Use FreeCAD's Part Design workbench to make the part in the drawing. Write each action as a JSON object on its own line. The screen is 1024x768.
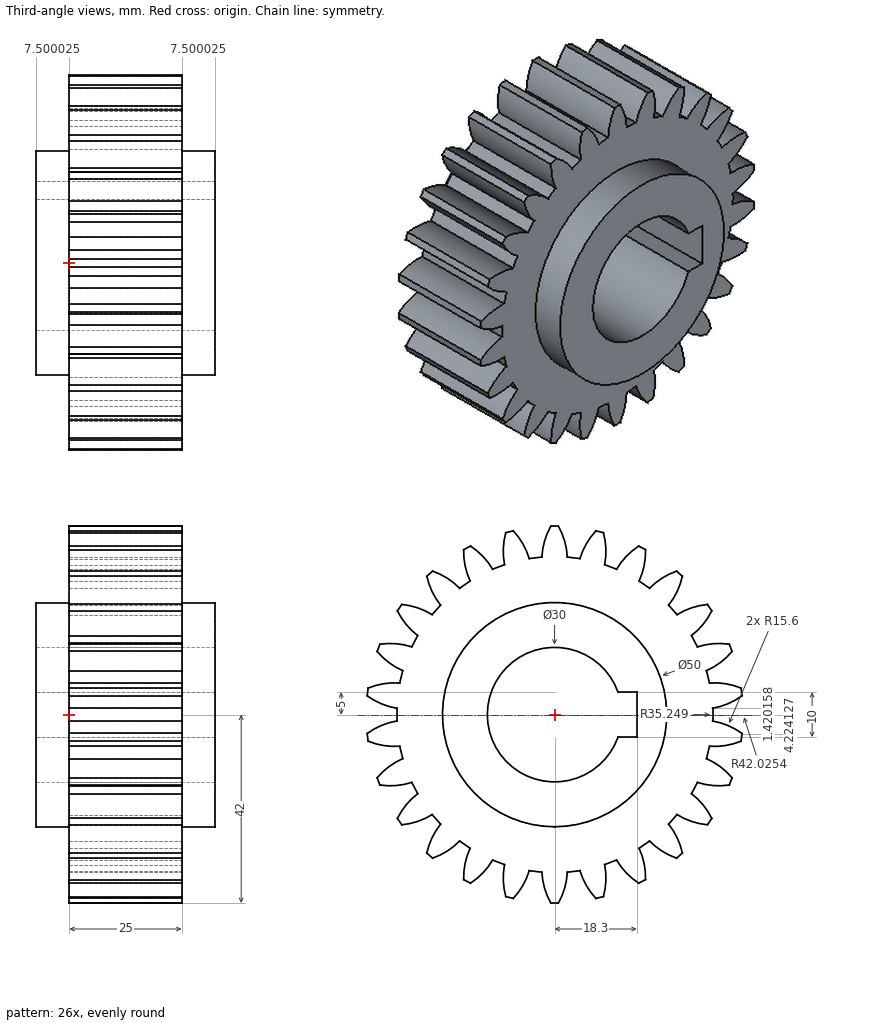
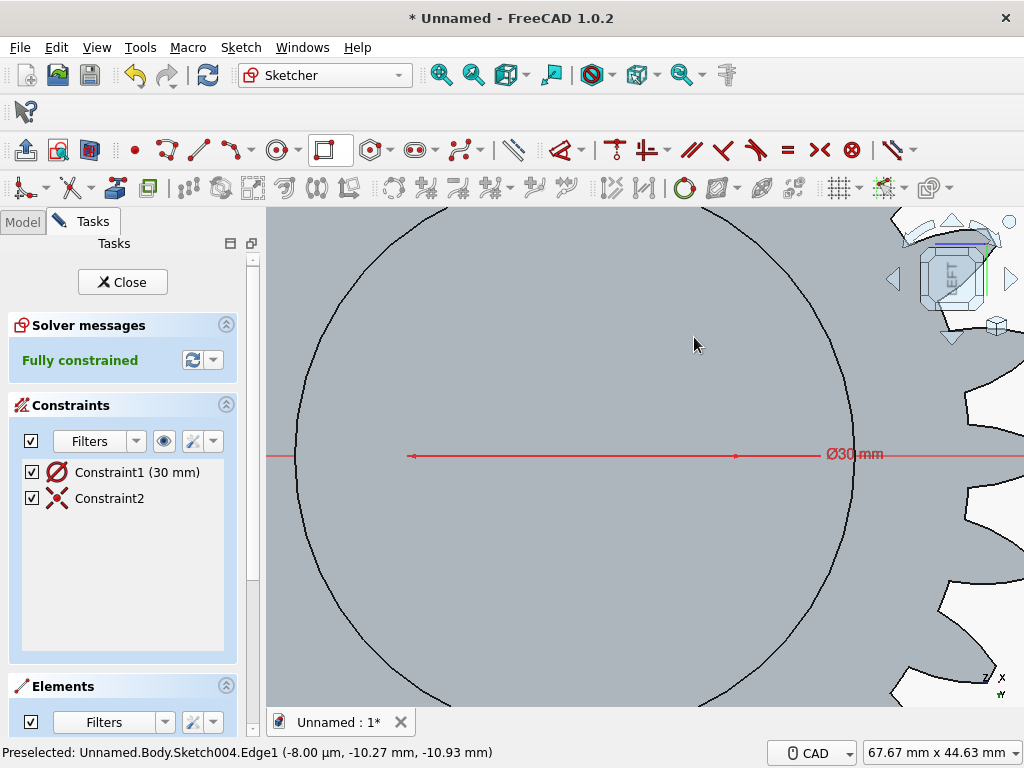
{"action": "left_click", "coordinate": [123, 282]}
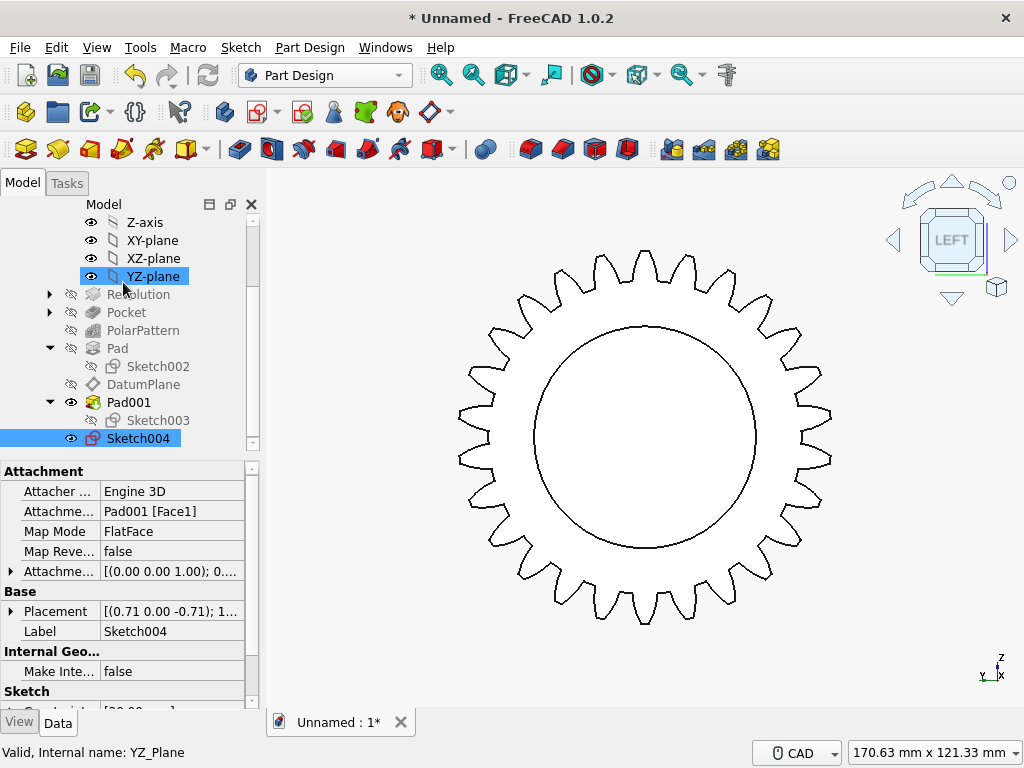
{"action": "left_click", "coordinate": [240, 150]}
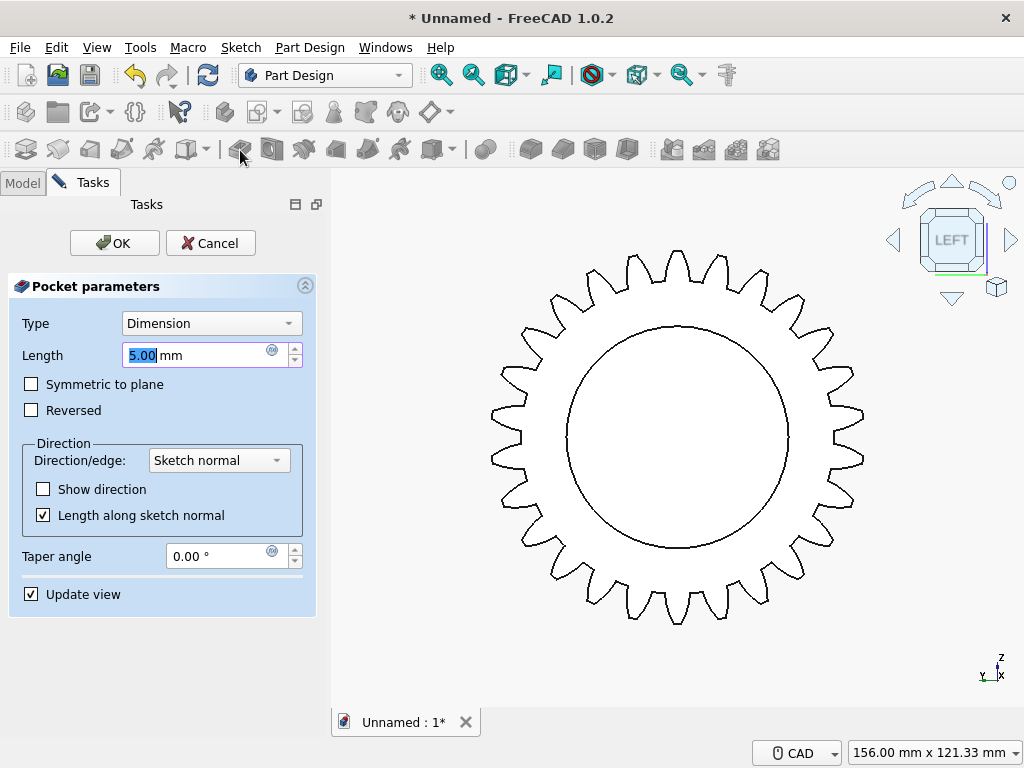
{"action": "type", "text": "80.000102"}
{"action": "key", "text": "Tab"}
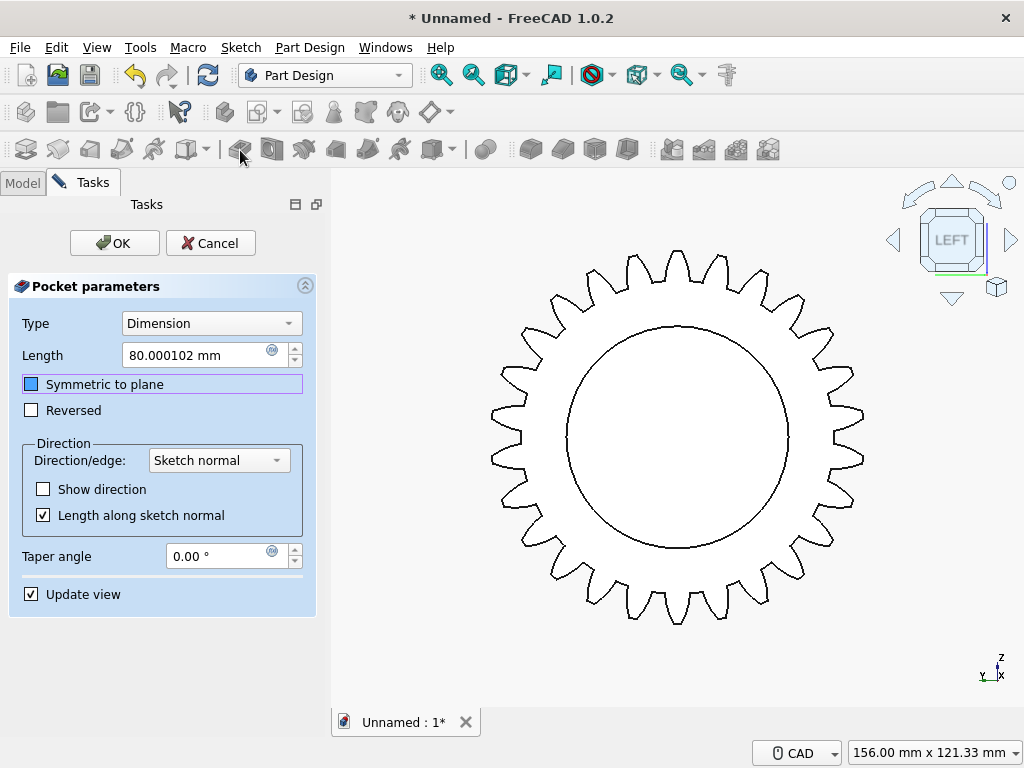
{"action": "left_click", "coordinate": [30, 384]}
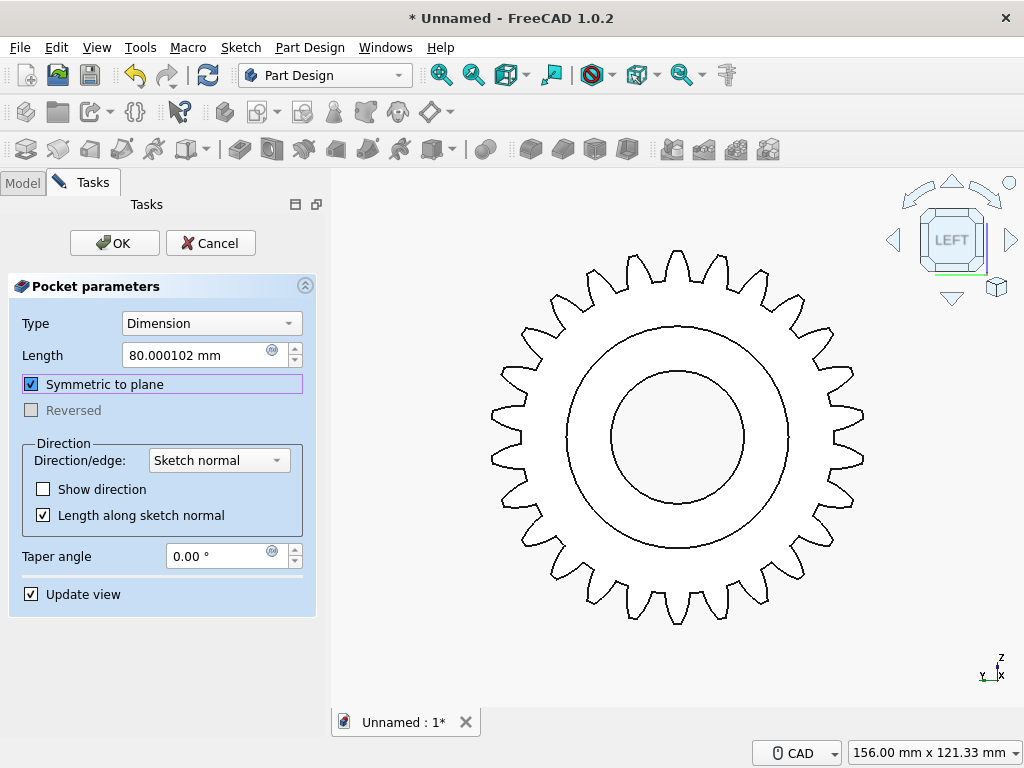
{"action": "left_click", "coordinate": [115, 243]}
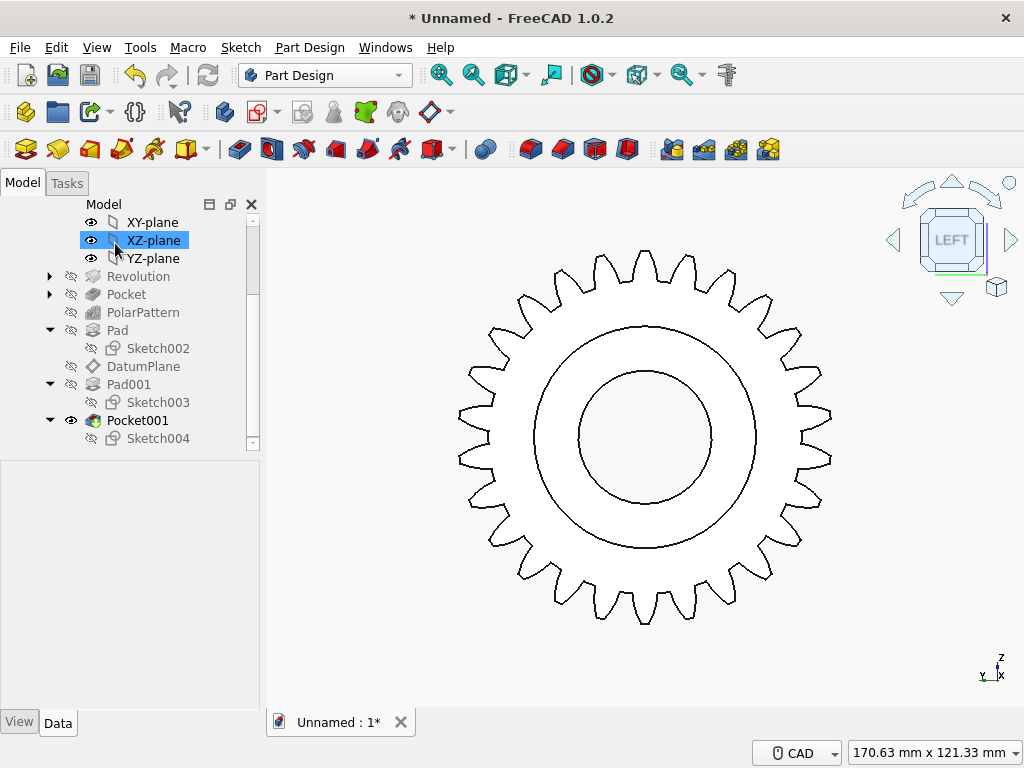
{"action": "left_click", "coordinate": [258, 112]}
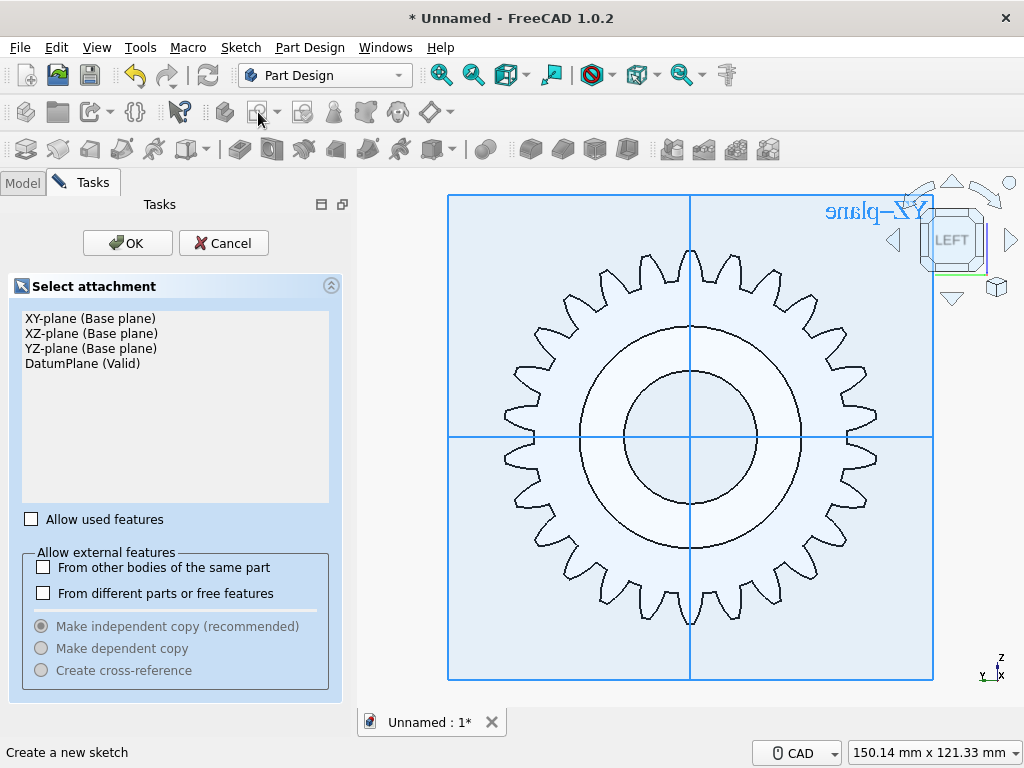
{"action": "left_click", "coordinate": [82, 348]}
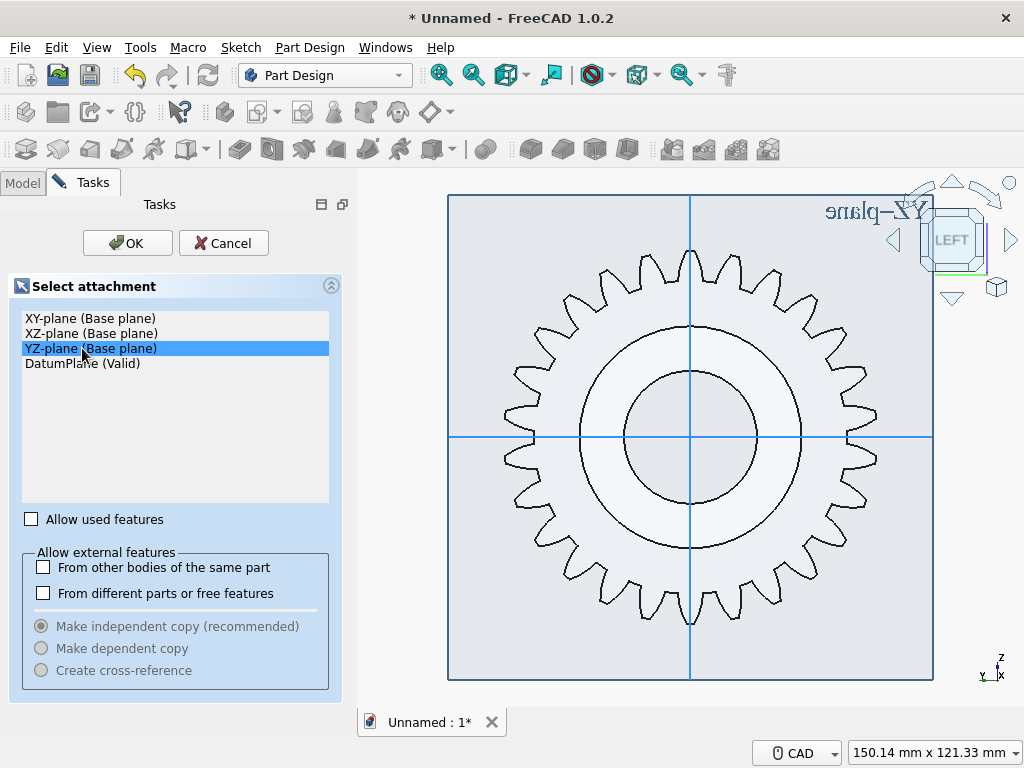
{"action": "left_click", "coordinate": [128, 243]}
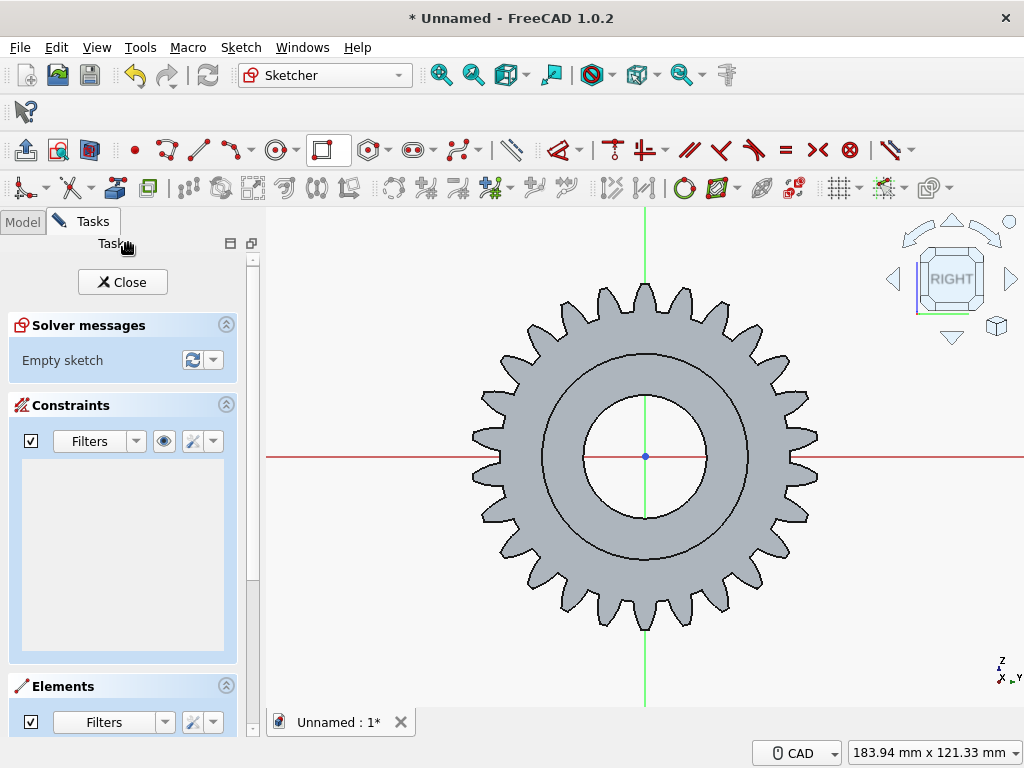
{"action": "left_click", "coordinate": [90, 150]}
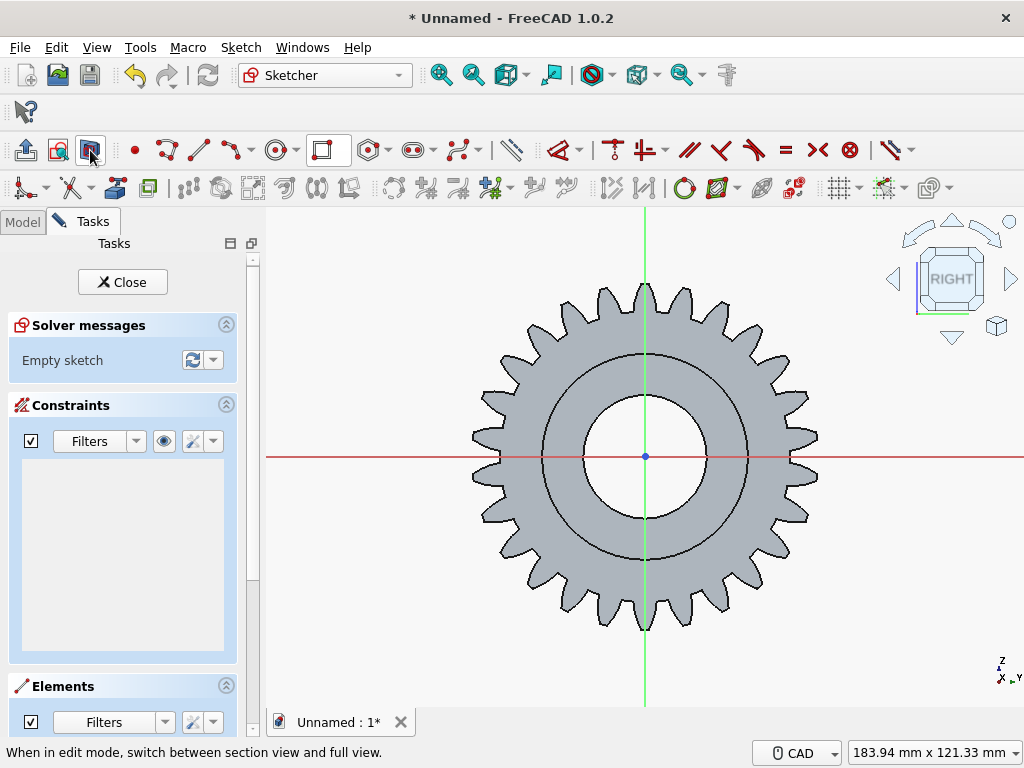
{"action": "scroll", "coordinate": [710, 457], "scroll_direction": "up", "scroll_amount": 8}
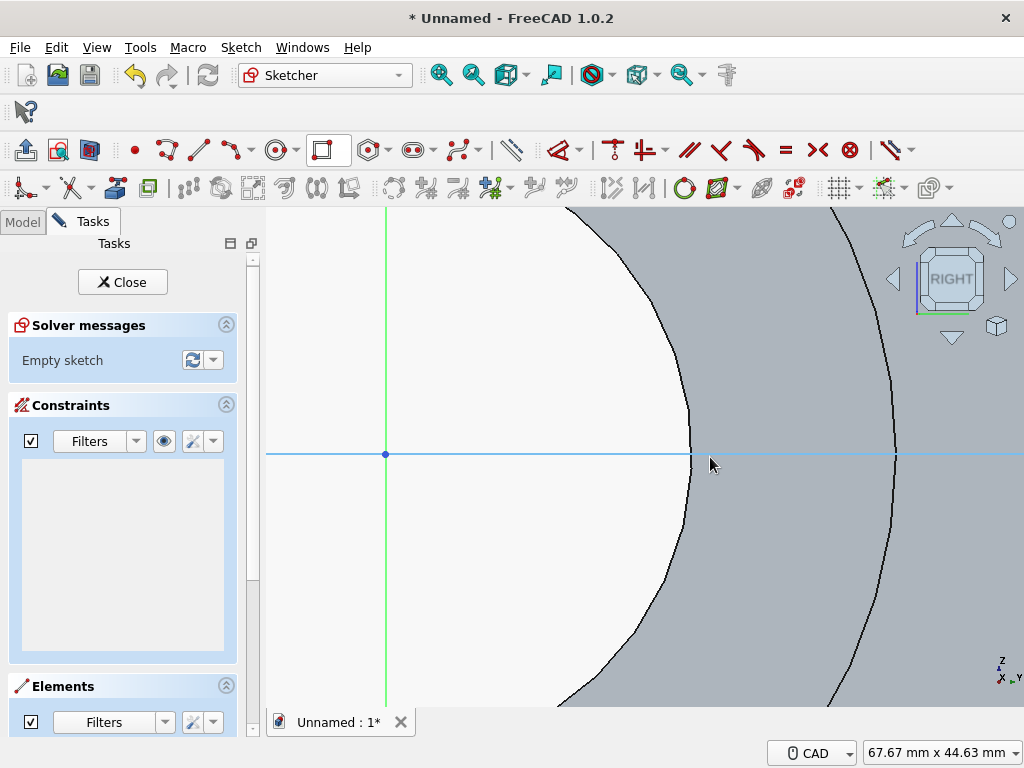
{"action": "left_click", "coordinate": [322, 150]}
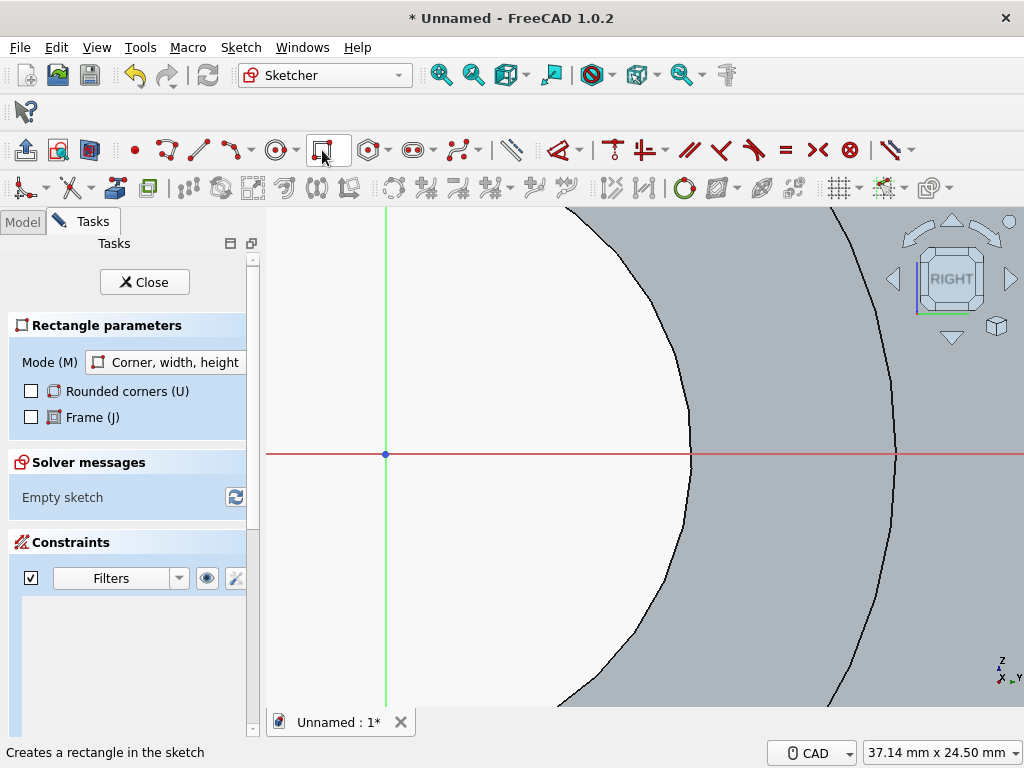
{"action": "left_click", "coordinate": [386, 352]}
{"action": "mouse_move", "coordinate": [759, 556]}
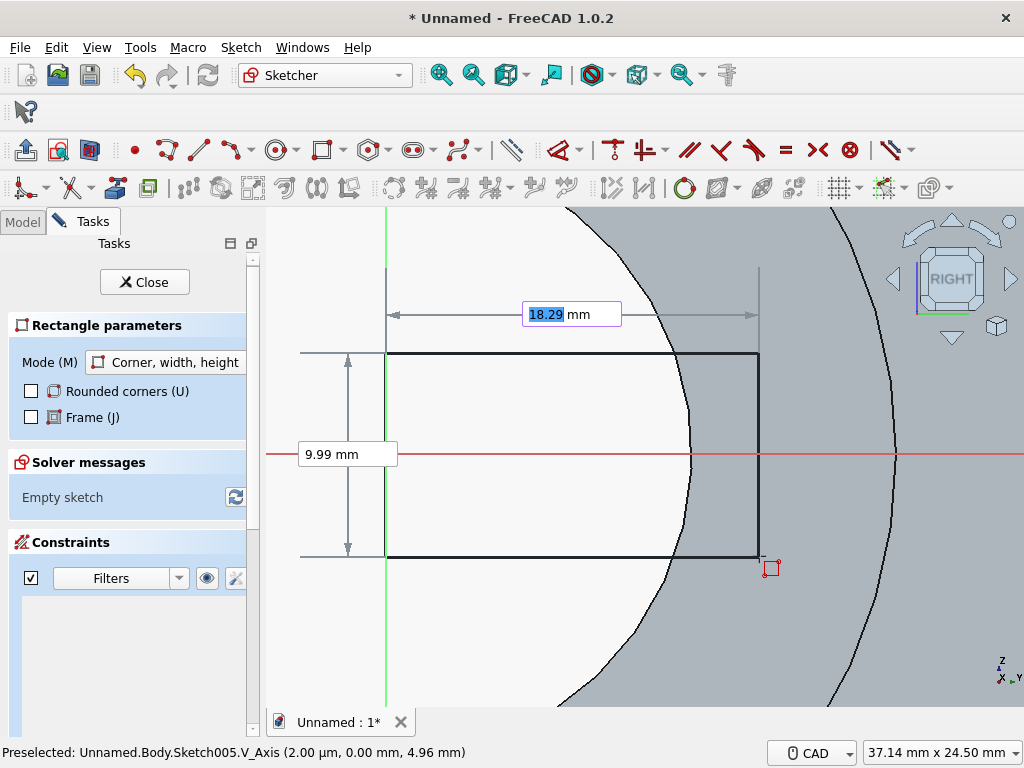
{"action": "type", "text": "18.3"}
{"action": "key", "text": "Tab"}
{"action": "type", "text": "10"}
{"action": "key", "text": "Return"}
{"action": "key", "text": "Escape"}